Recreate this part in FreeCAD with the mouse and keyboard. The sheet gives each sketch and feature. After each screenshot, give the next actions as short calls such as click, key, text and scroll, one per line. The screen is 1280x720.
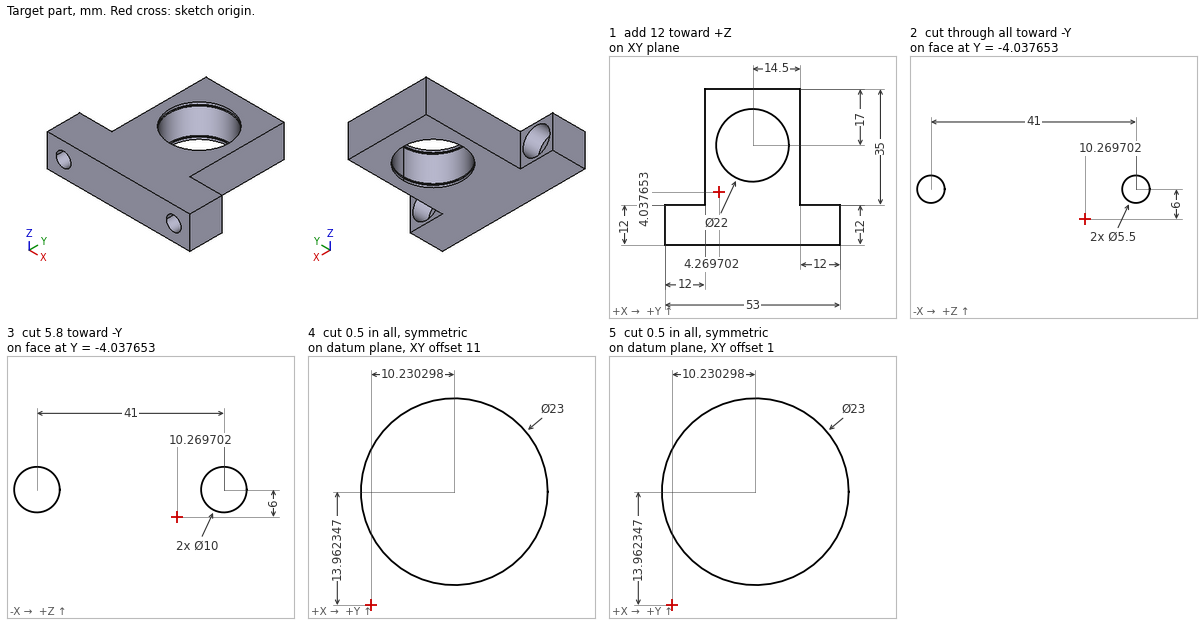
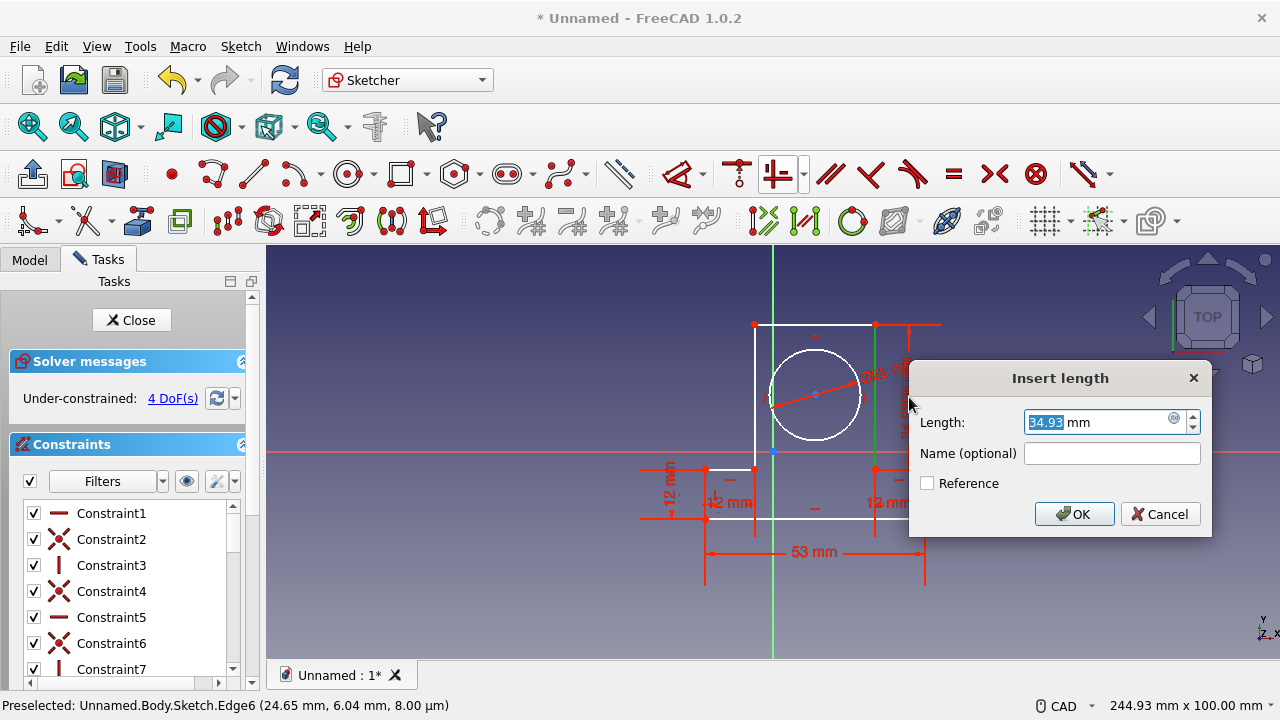
text(35)
key(Return)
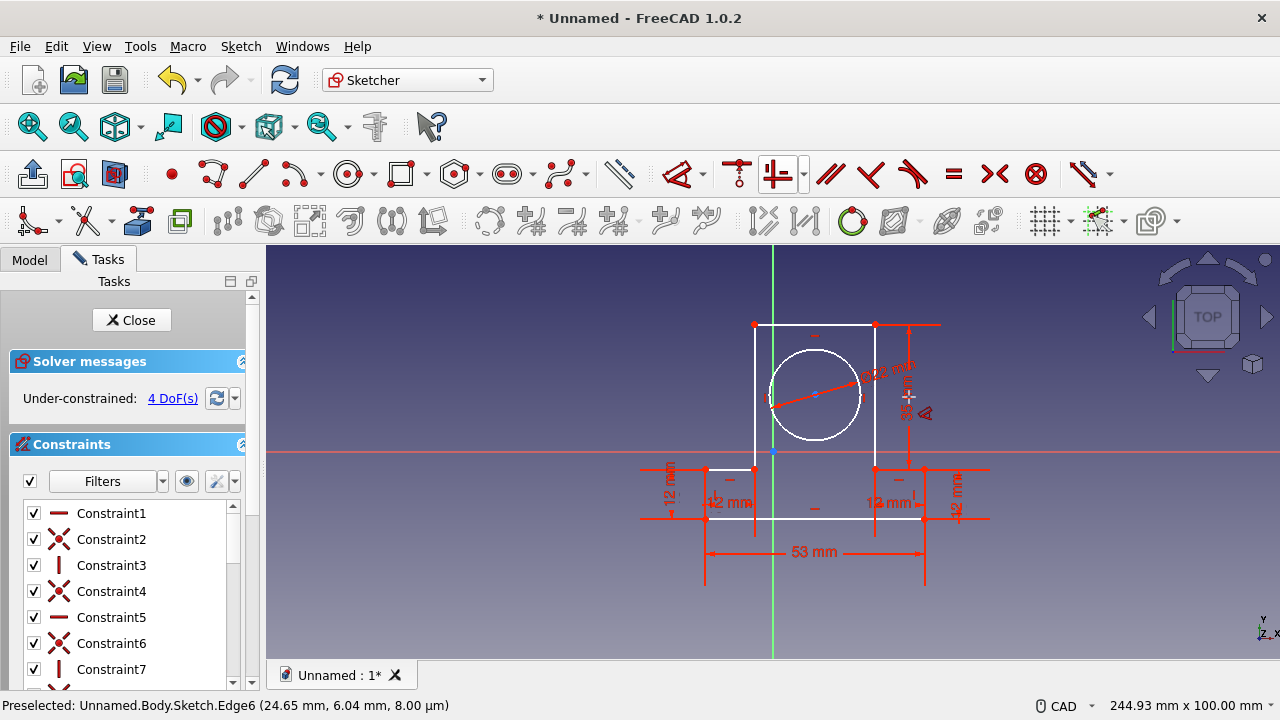
click(875, 325)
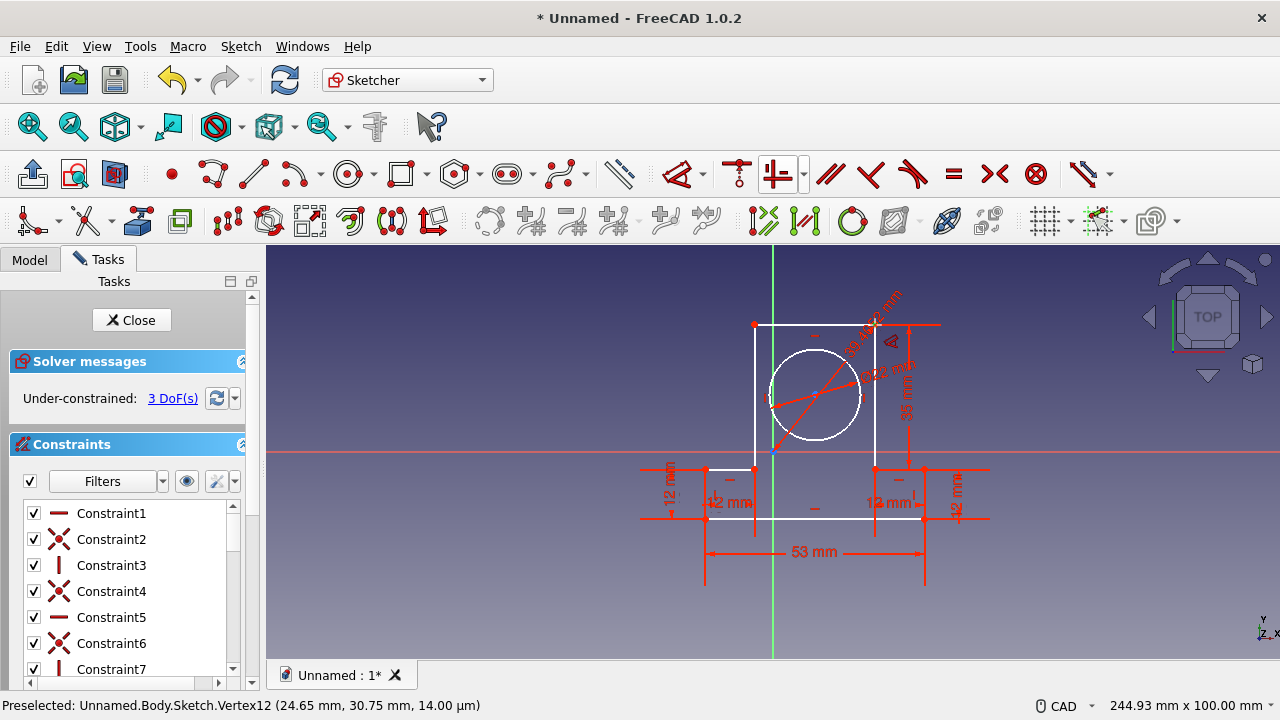
click(815, 395)
click(909, 344)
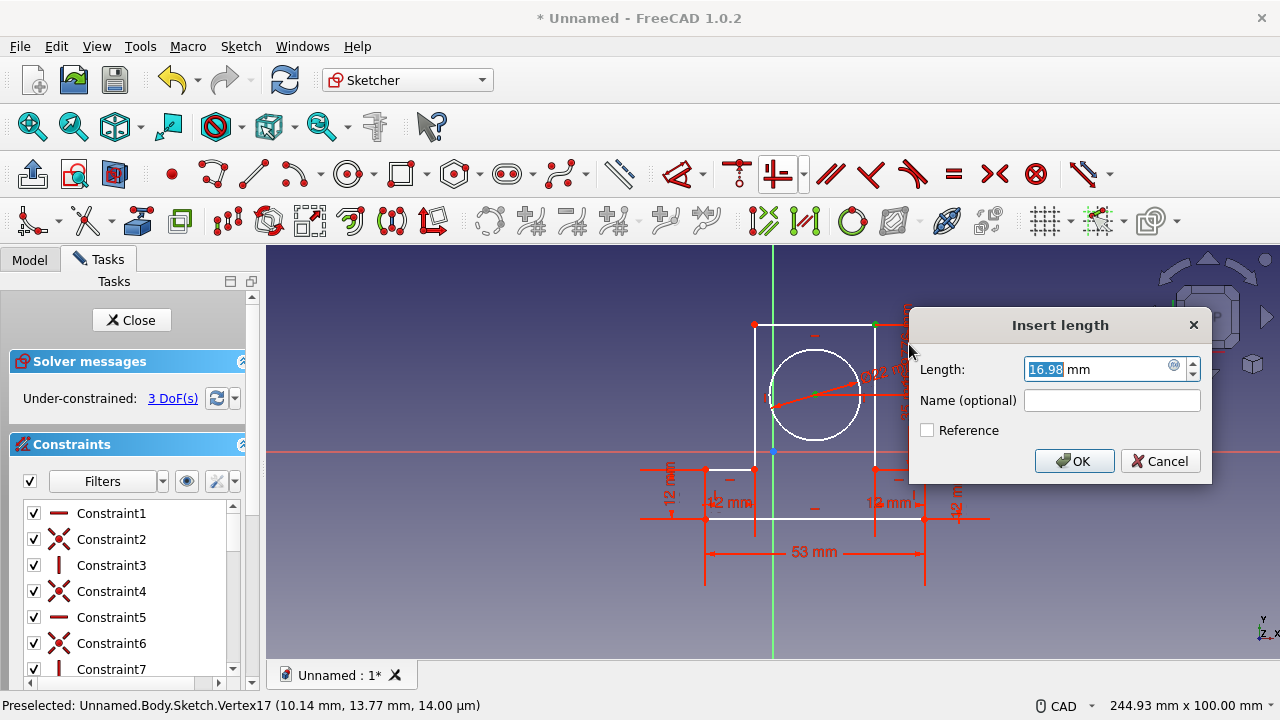
text(17)
key(Return)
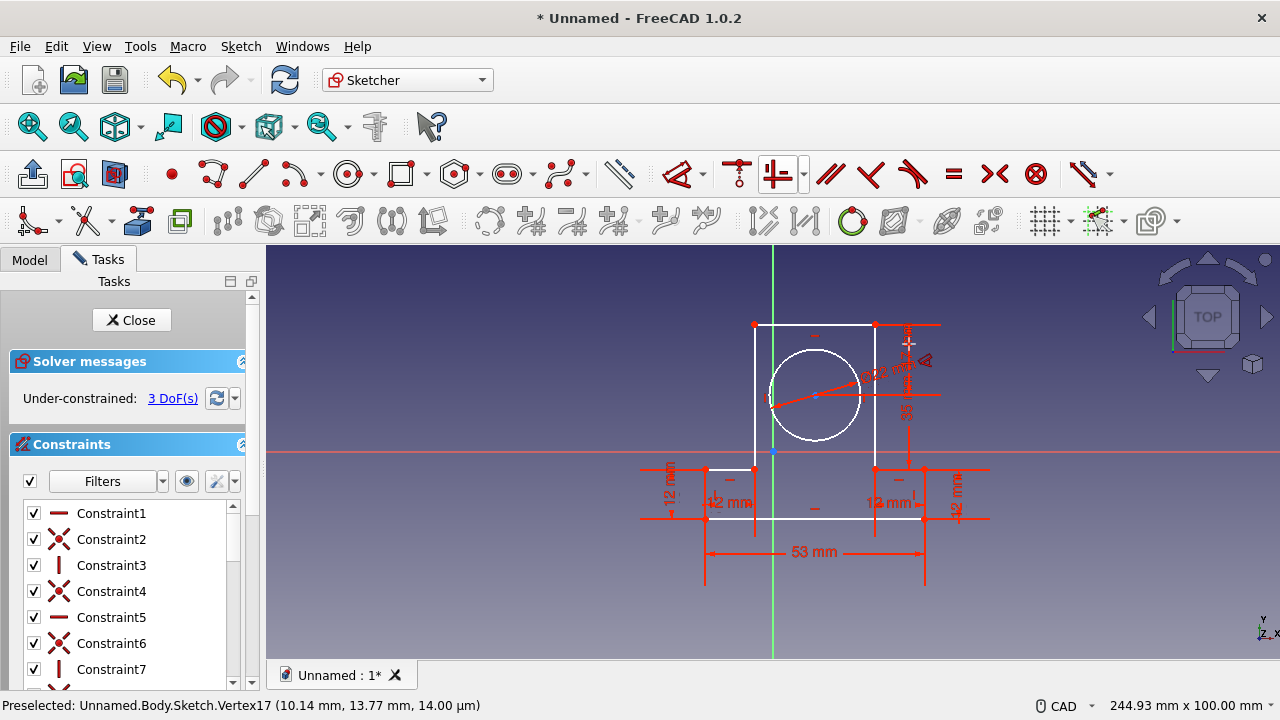
click(875, 325)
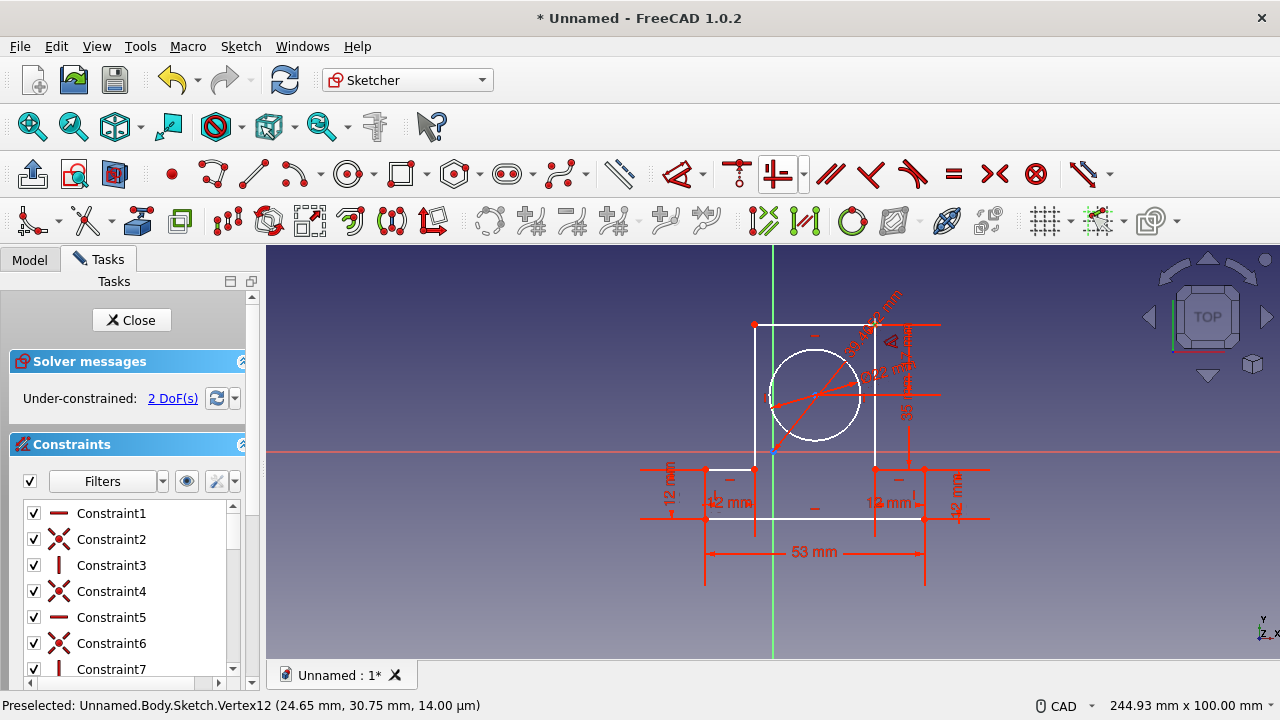
click(815, 395)
click(845, 291)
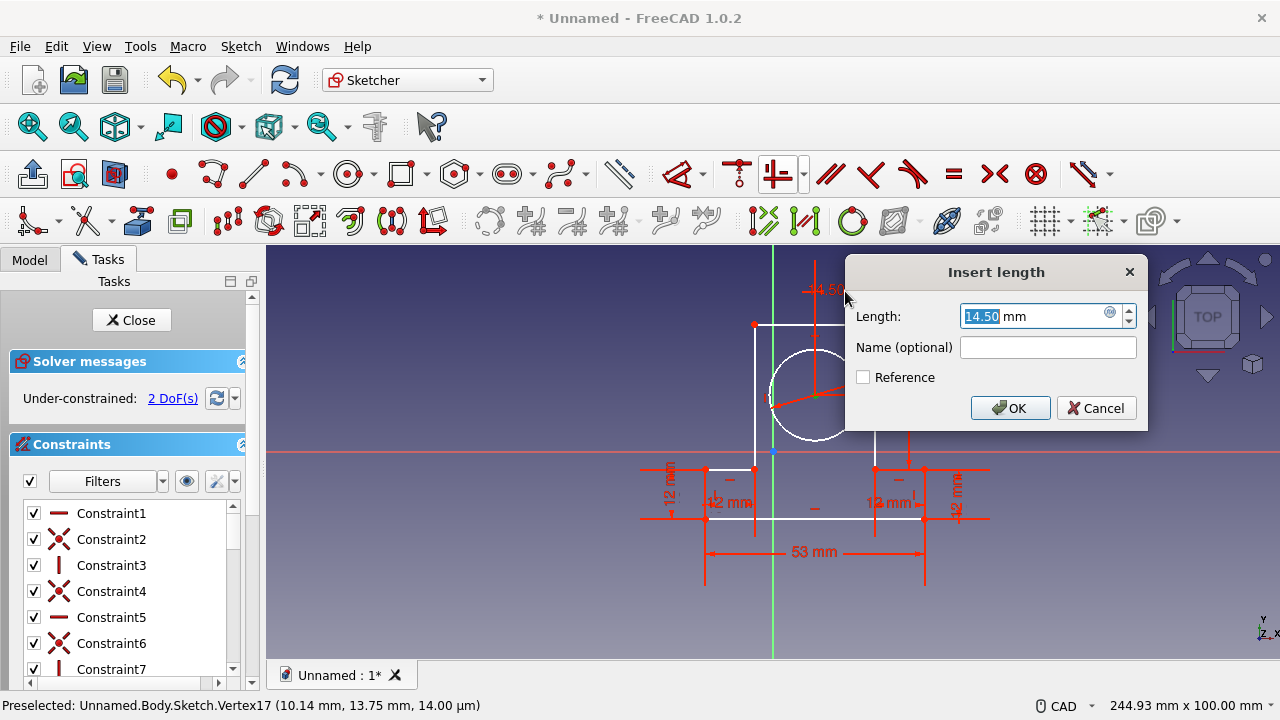
text(14.5)
key(Return)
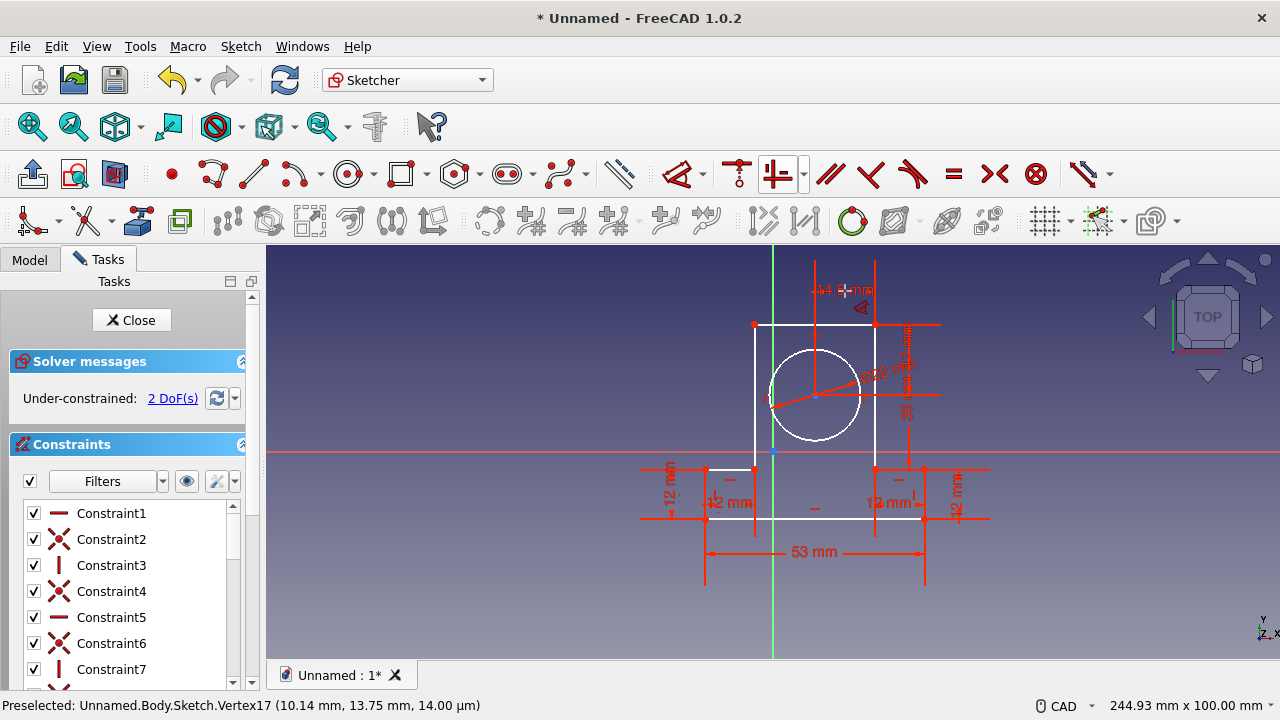
scroll(755, 470, up, 5)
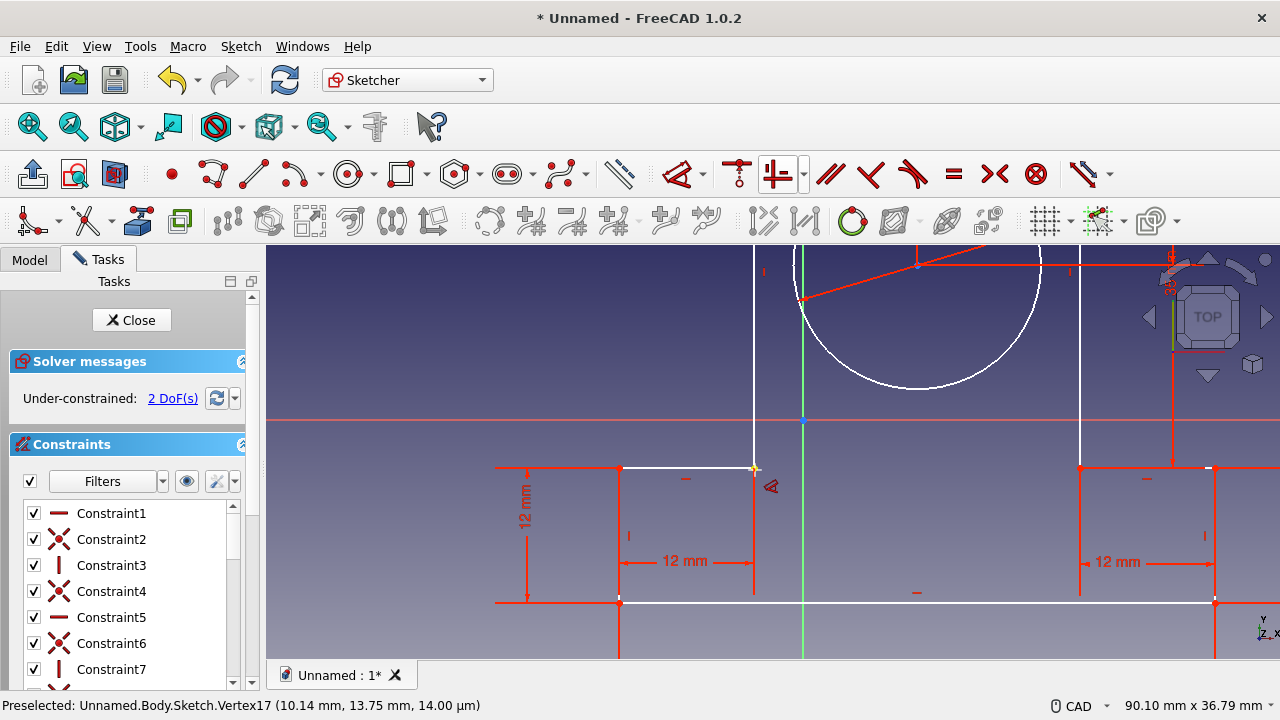
click(754, 468)
click(779, 502)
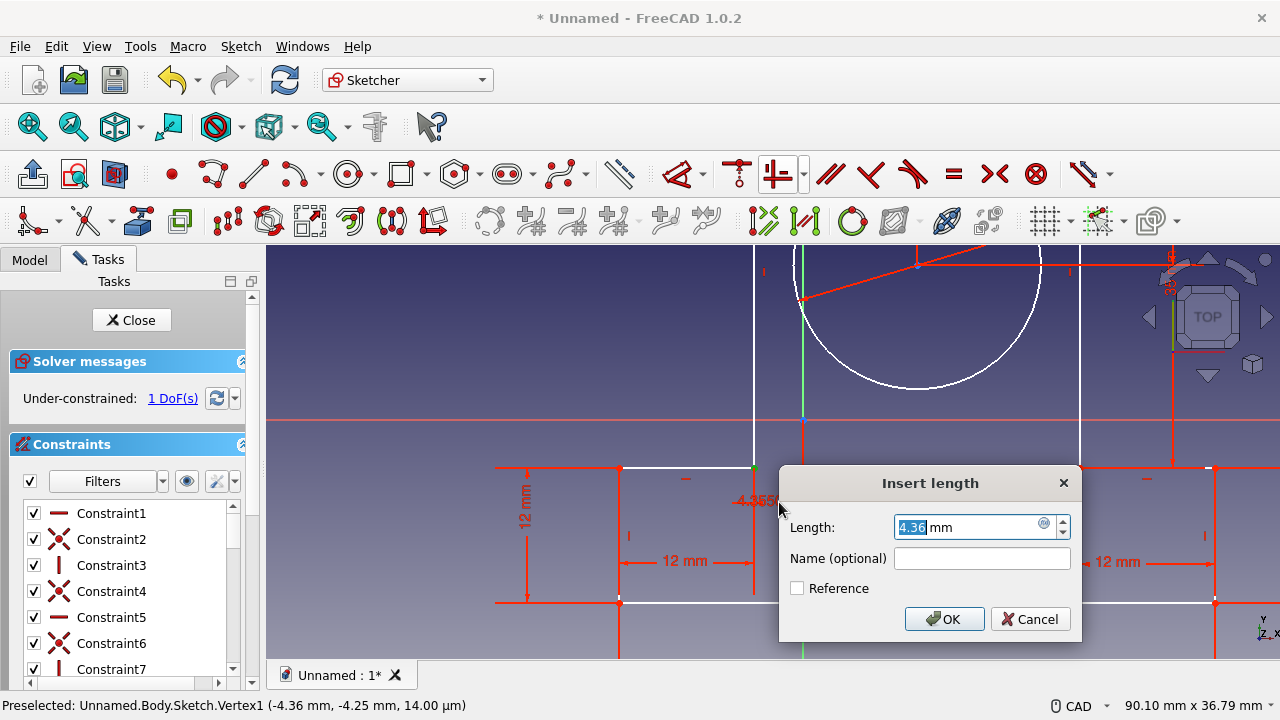
text(4.269702)
key(Return)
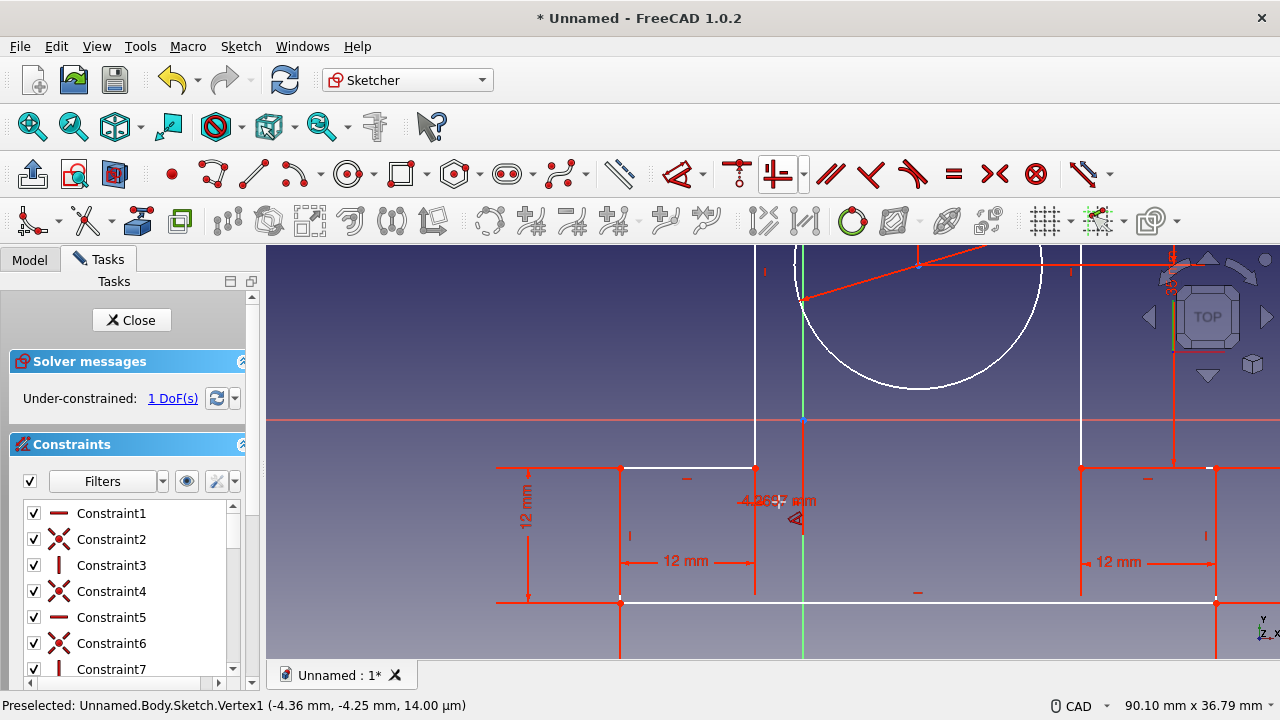
click(755, 468)
click(721, 444)